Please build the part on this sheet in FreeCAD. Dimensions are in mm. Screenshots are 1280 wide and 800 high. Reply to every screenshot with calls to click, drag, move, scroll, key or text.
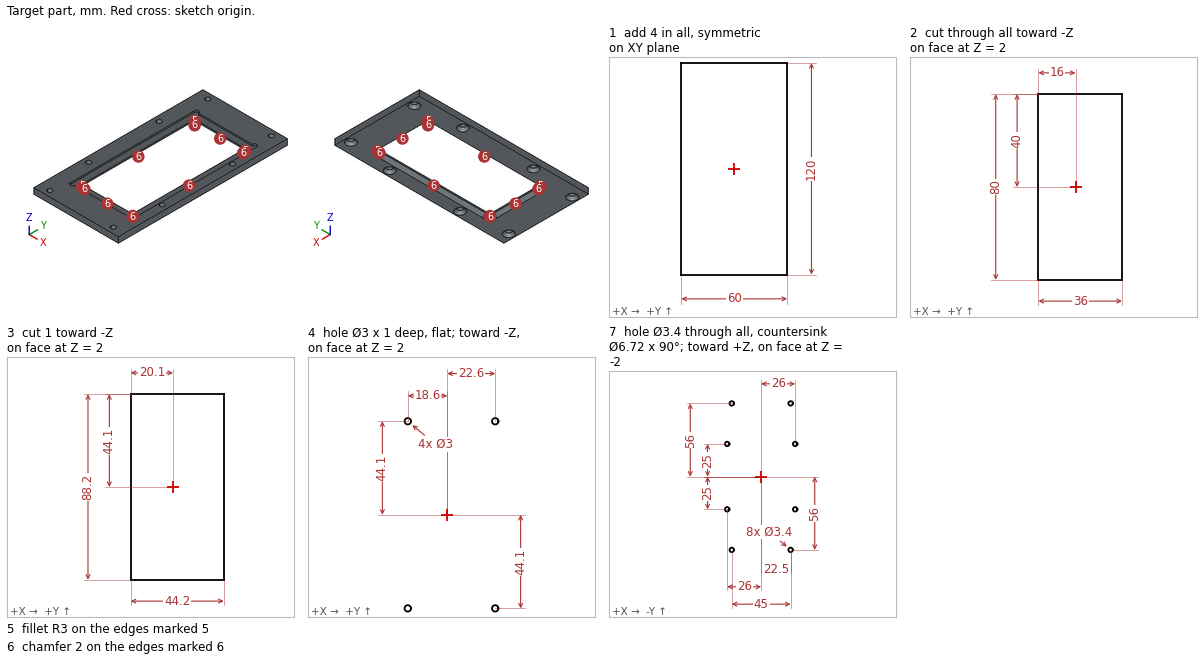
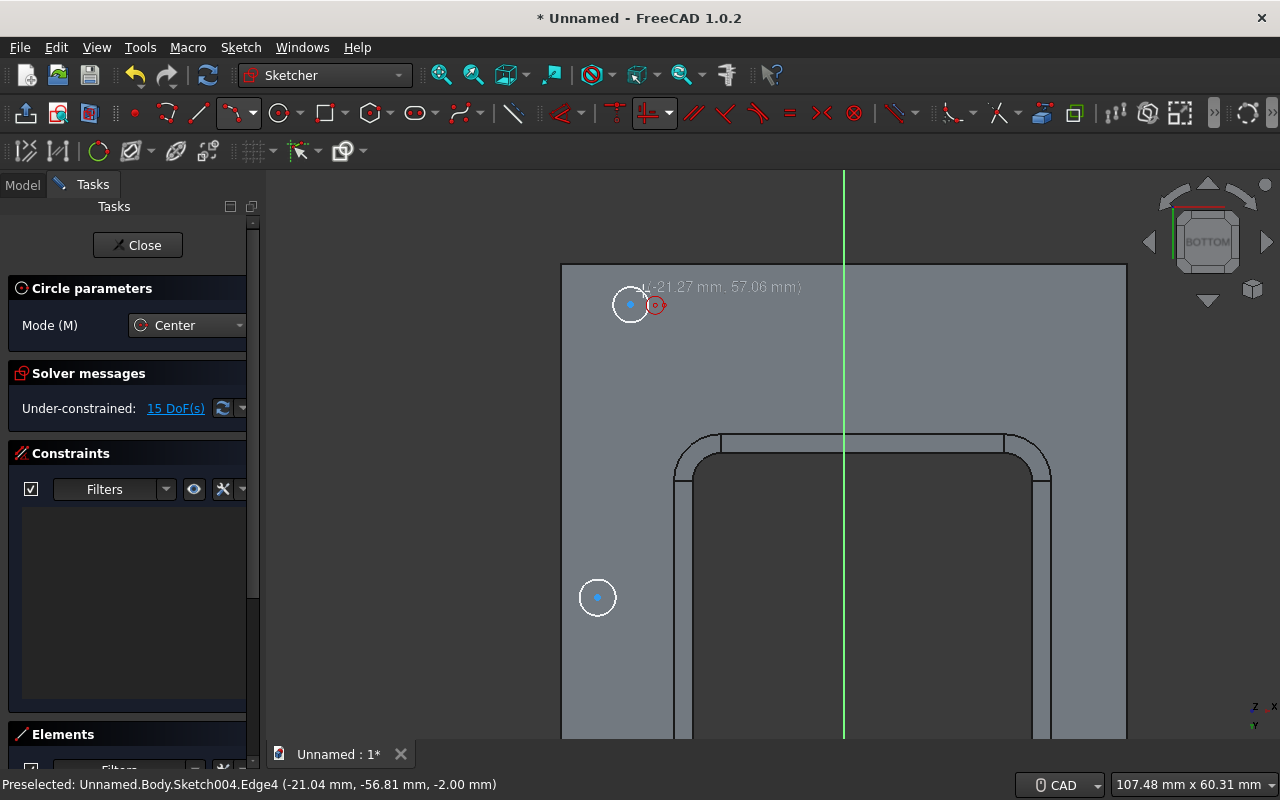
scroll(1056, 302, up, 2)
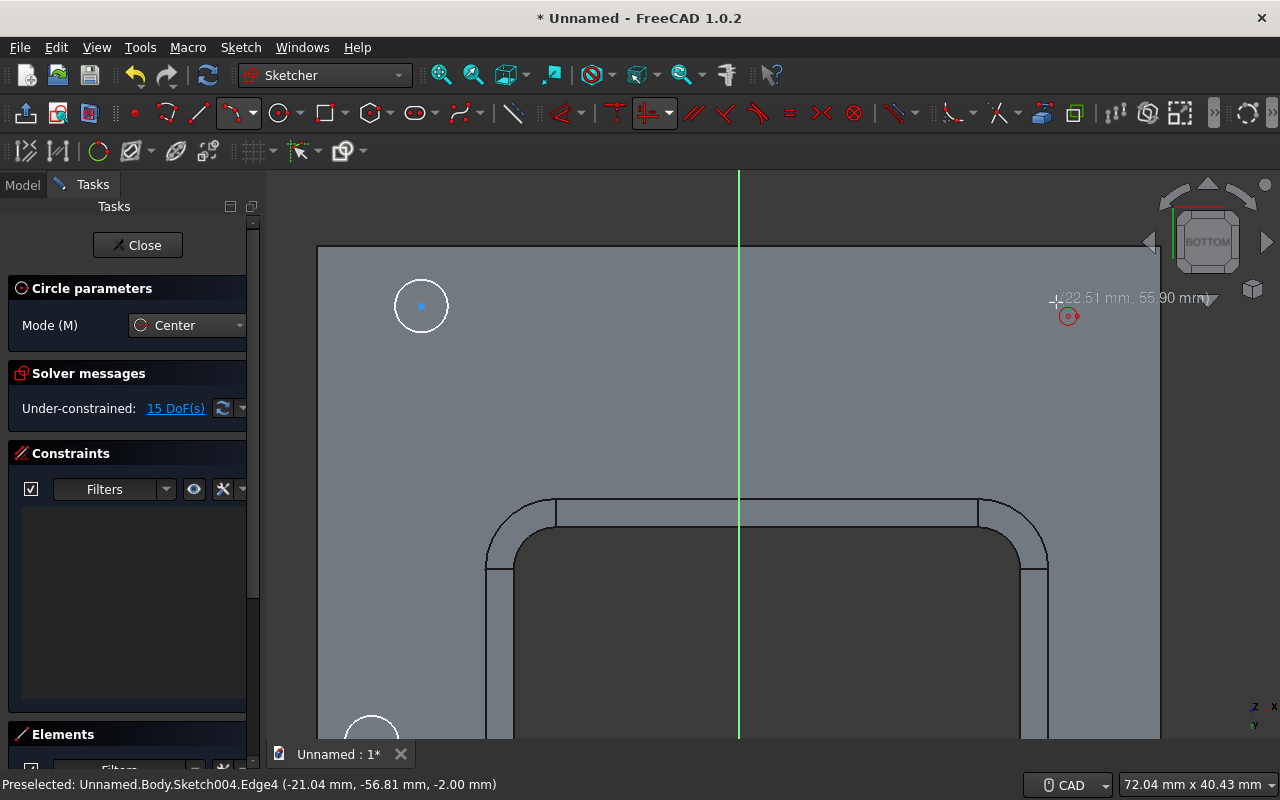
scroll(696, 294, down, 8)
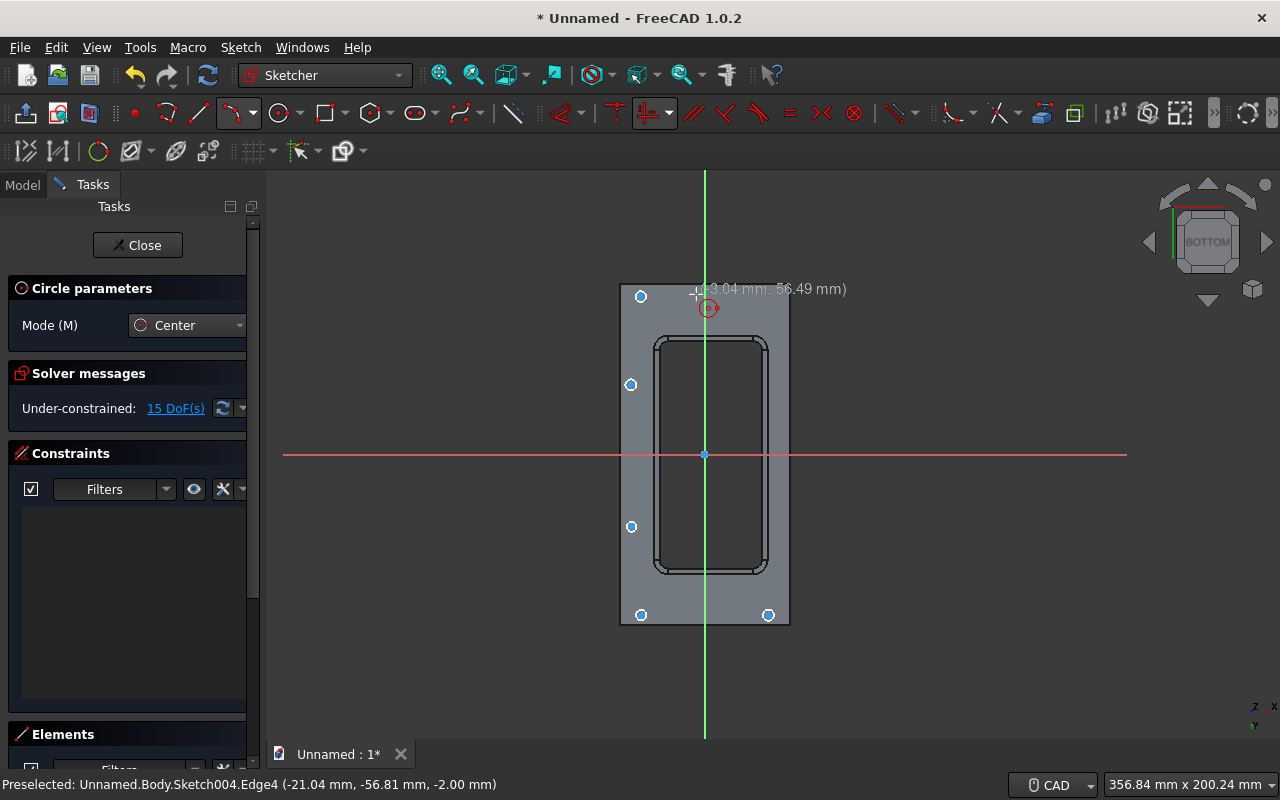
click(769, 296)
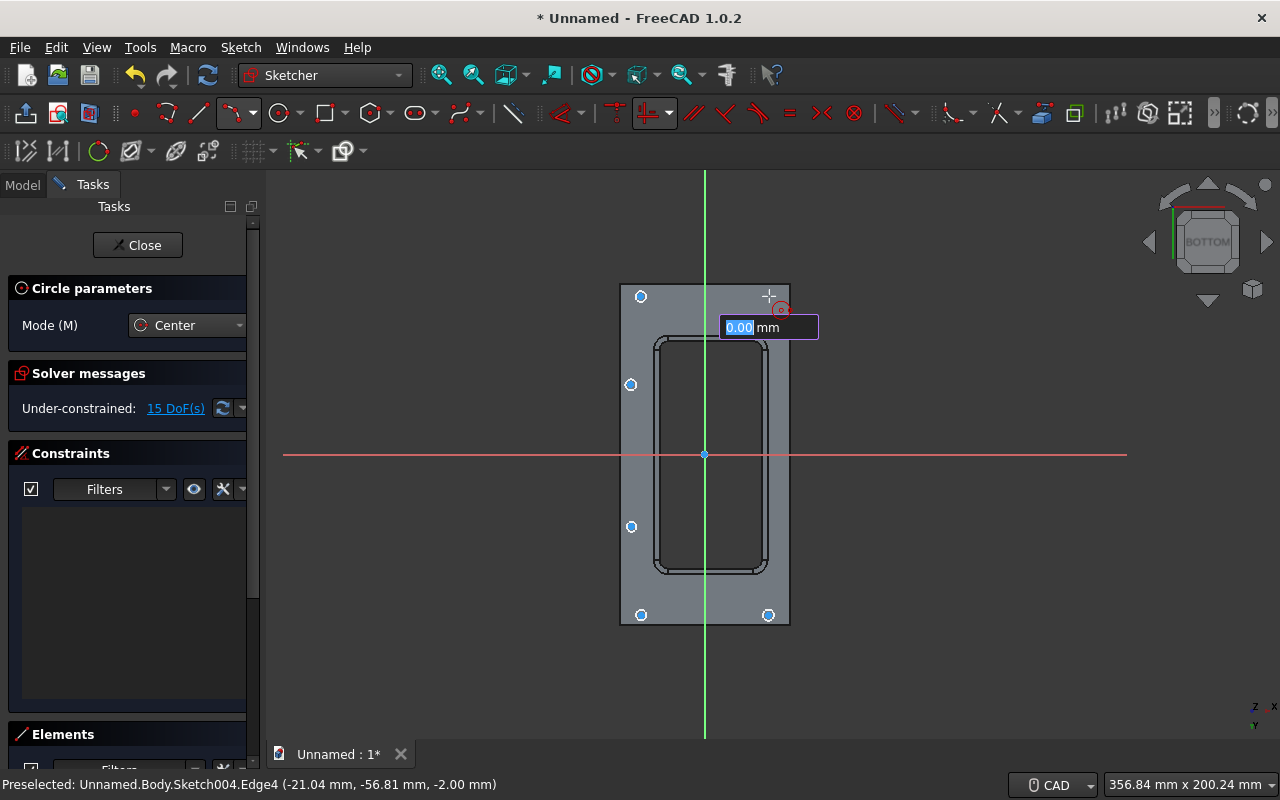
scroll(772, 292, up, 6)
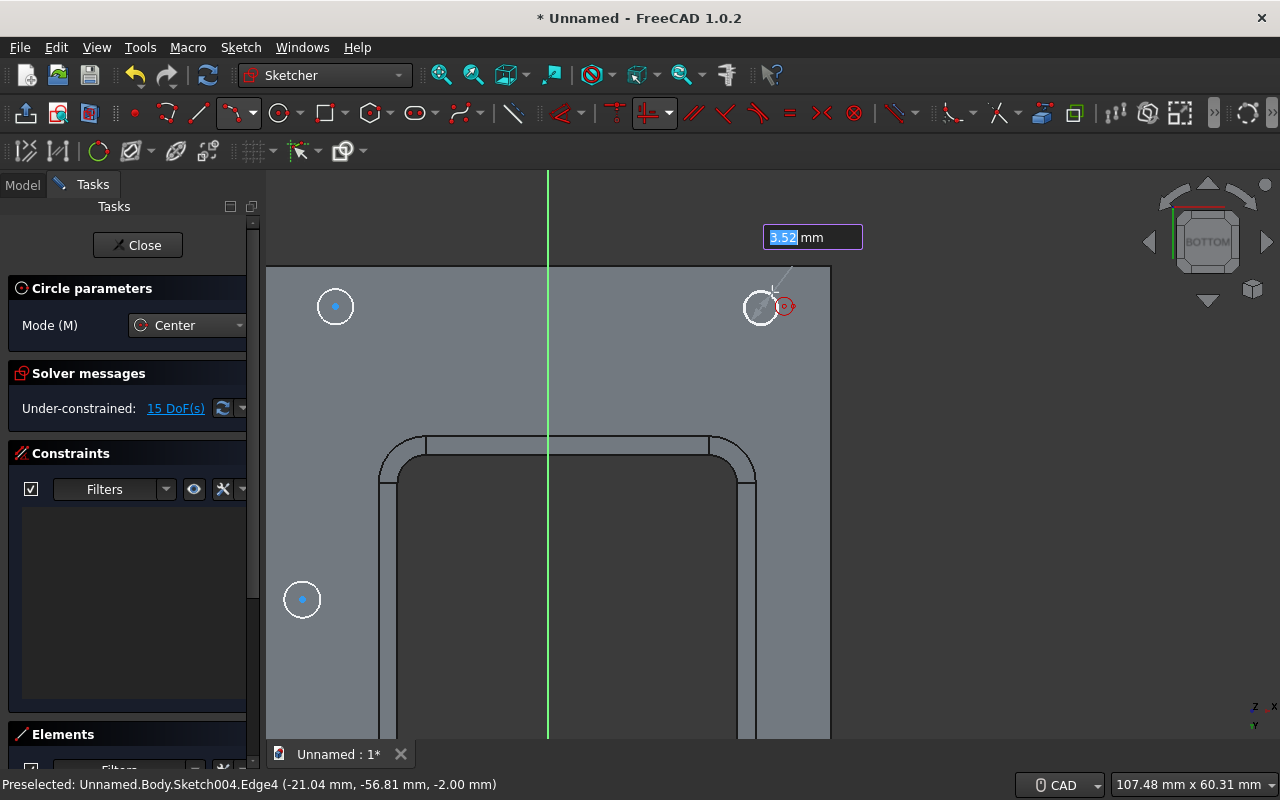
click(772, 293)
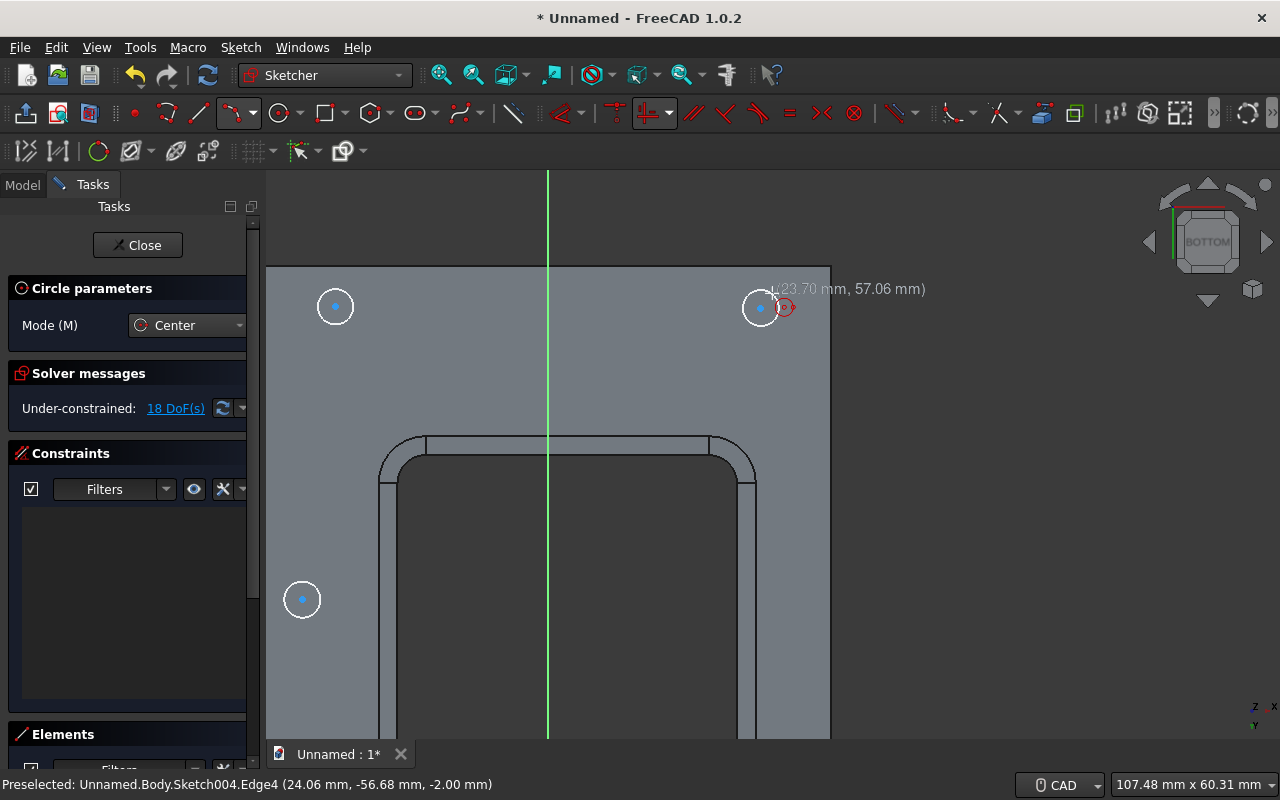
scroll(794, 597, up, 2)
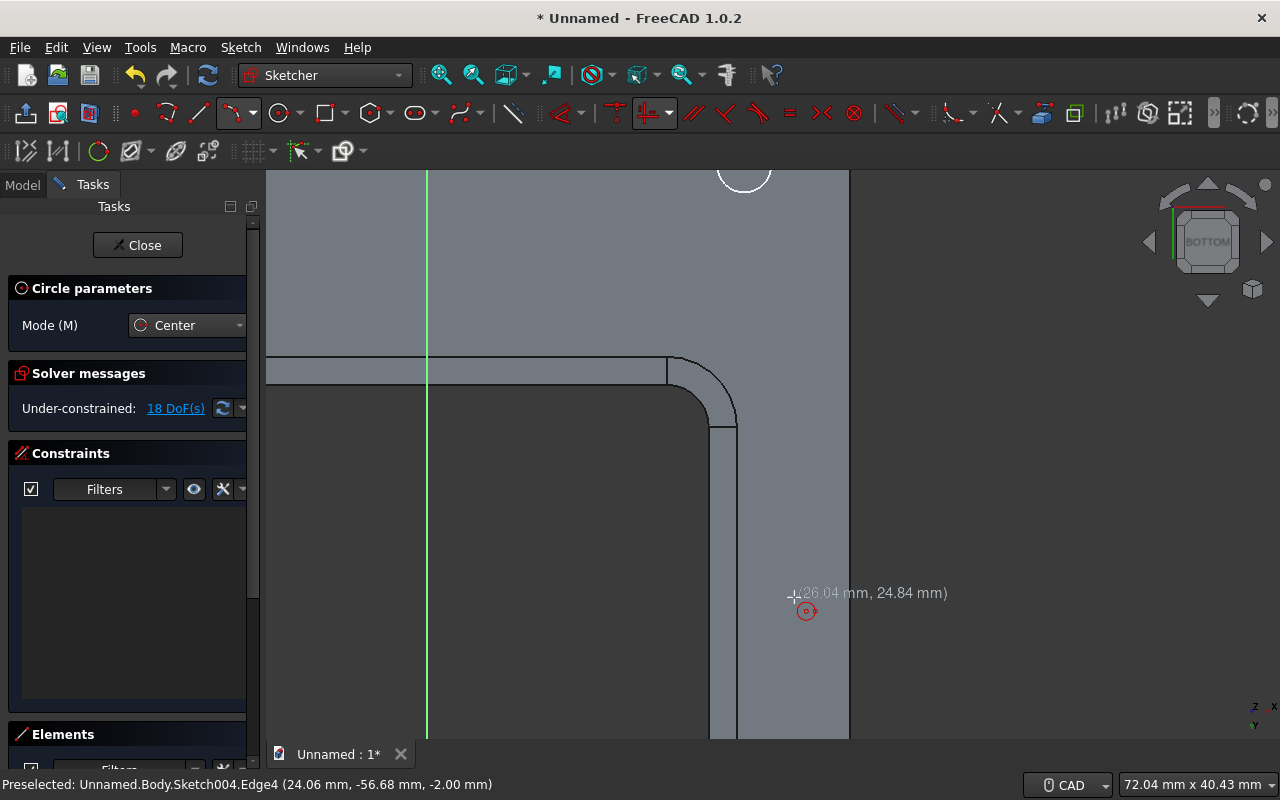
scroll(775, 330, down, 8)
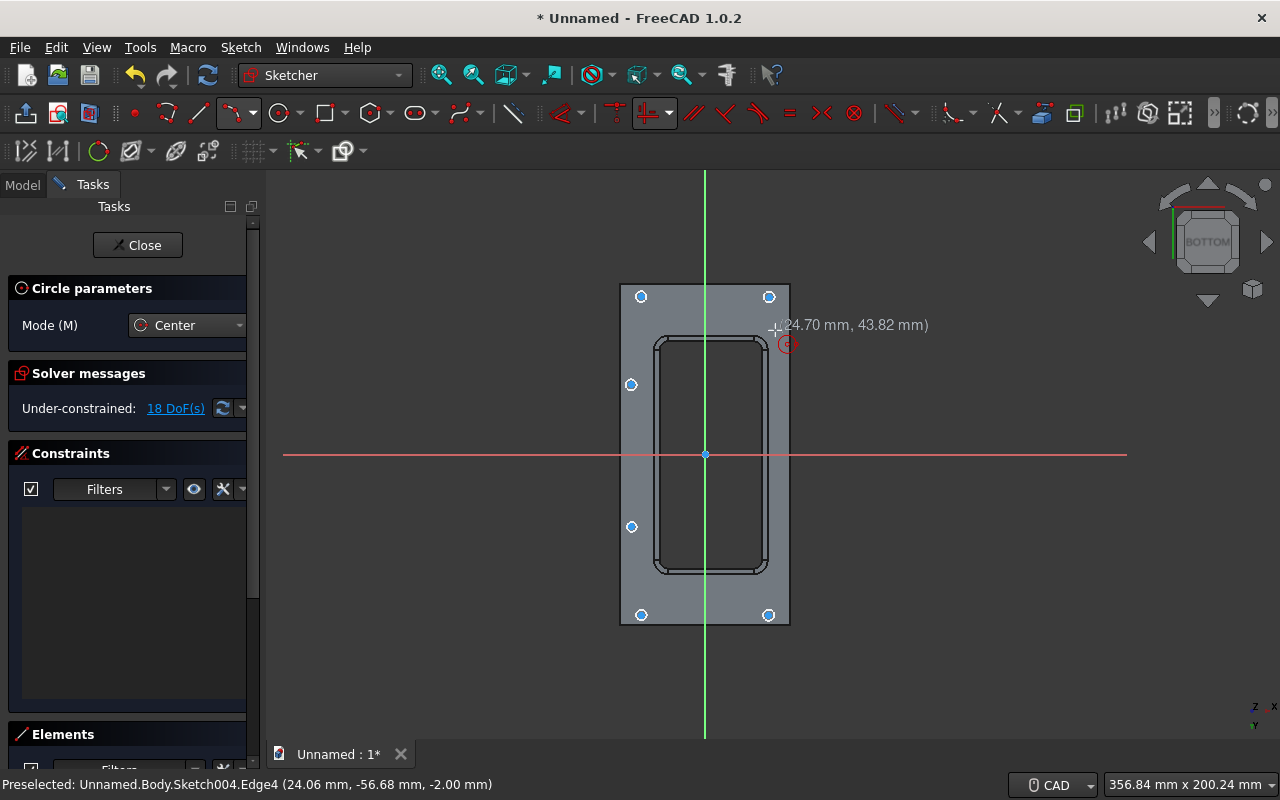
click(779, 384)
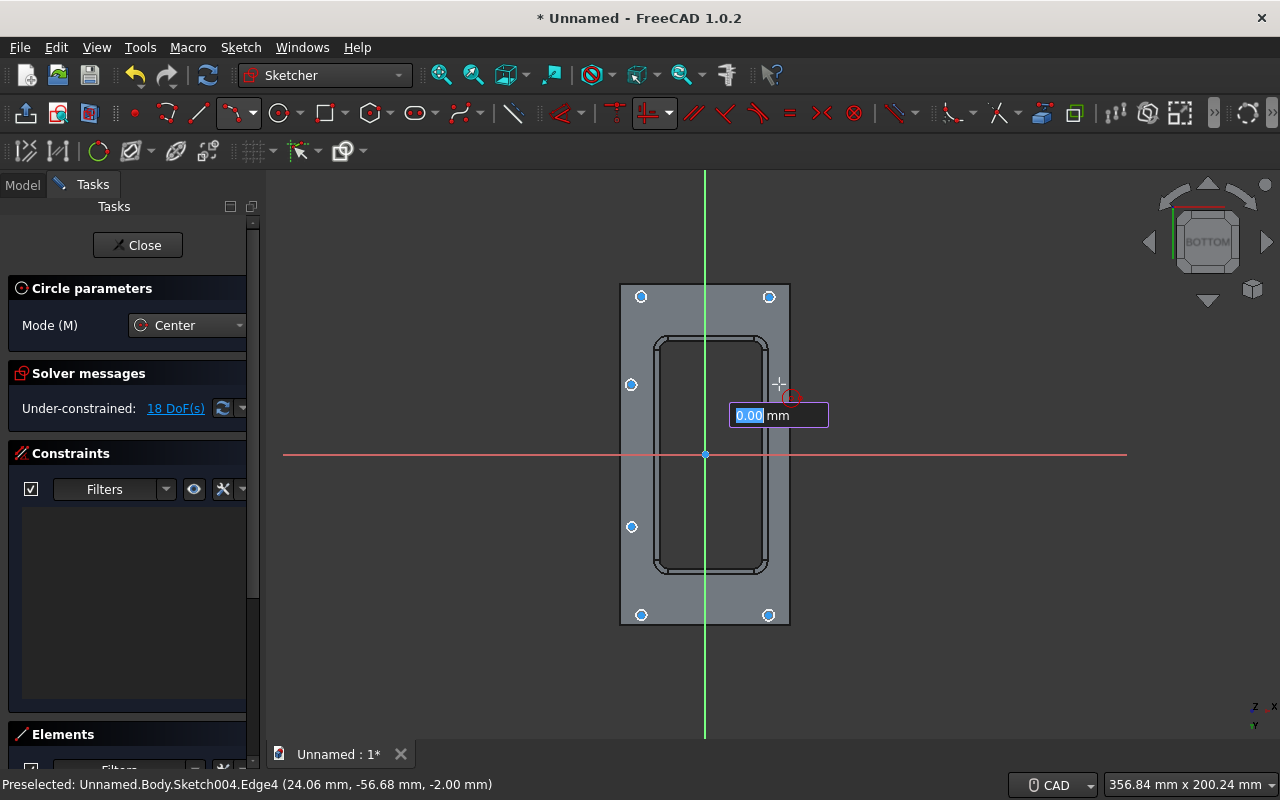
scroll(782, 380, up, 6)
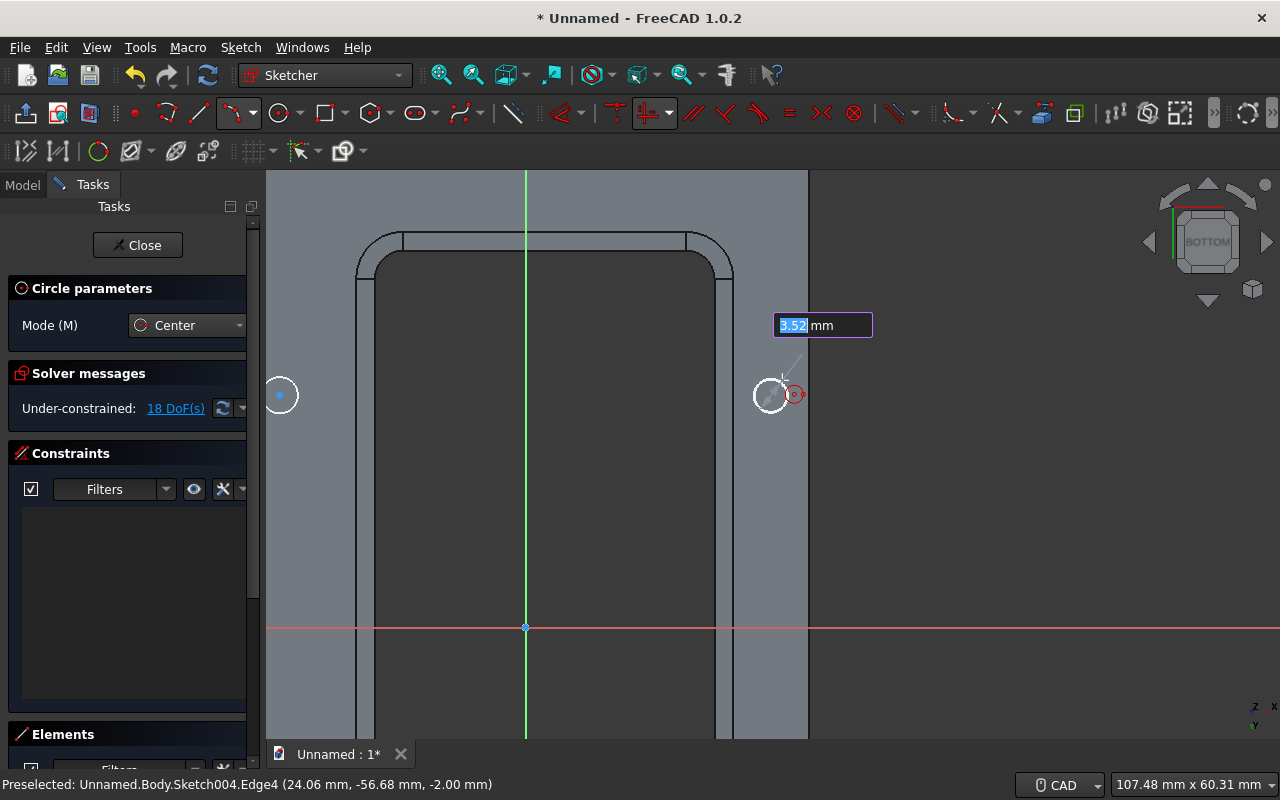
click(782, 381)